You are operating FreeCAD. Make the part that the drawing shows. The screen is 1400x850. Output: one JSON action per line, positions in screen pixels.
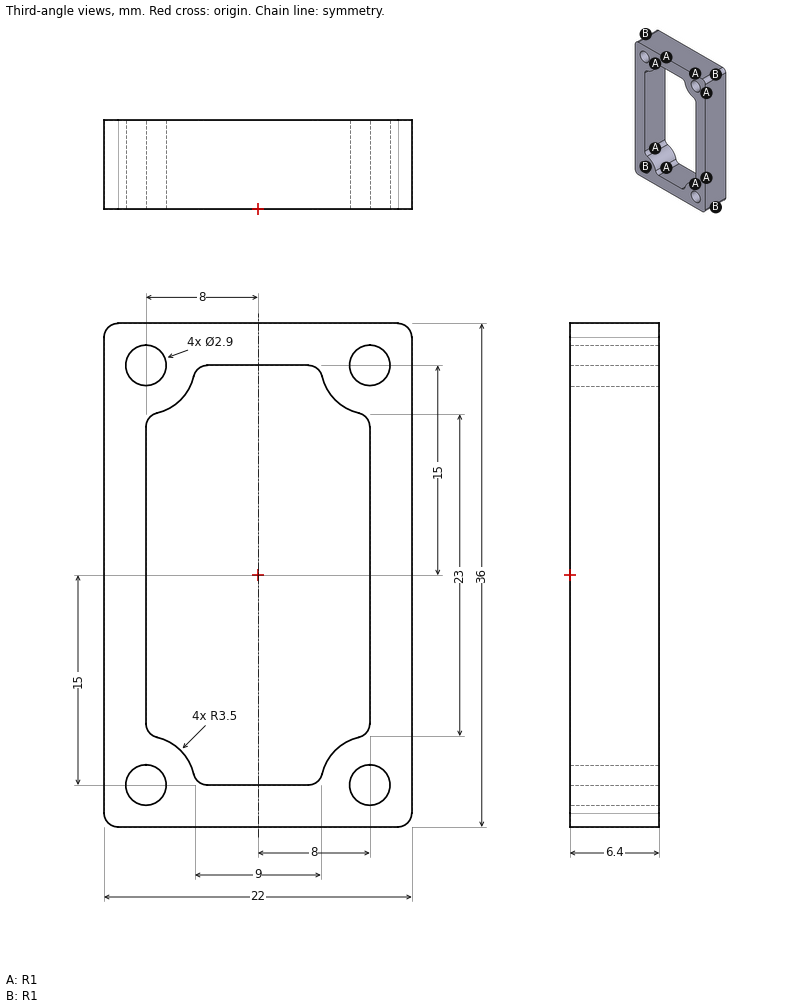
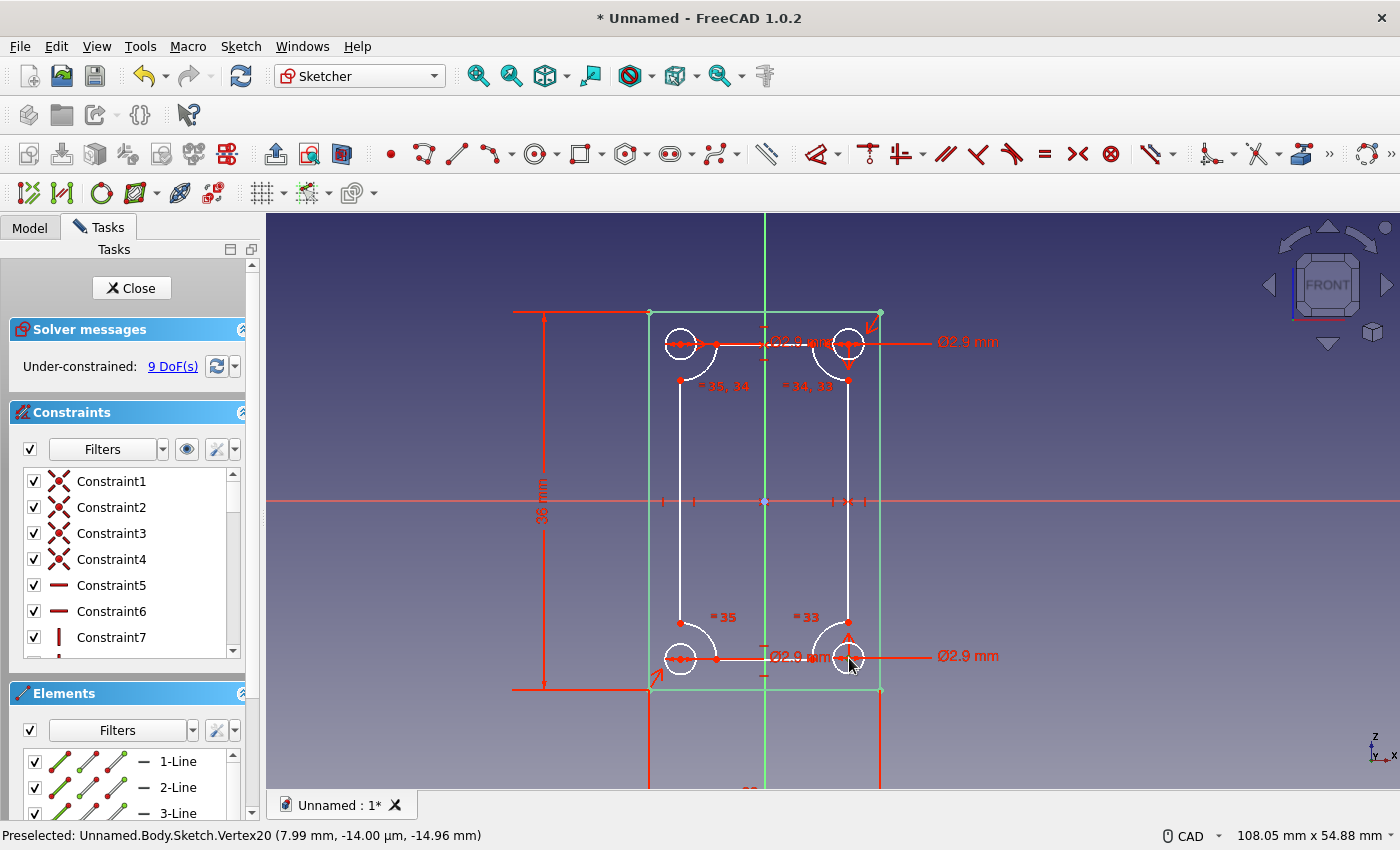
{"action": "left_click", "coordinate": [680, 659]}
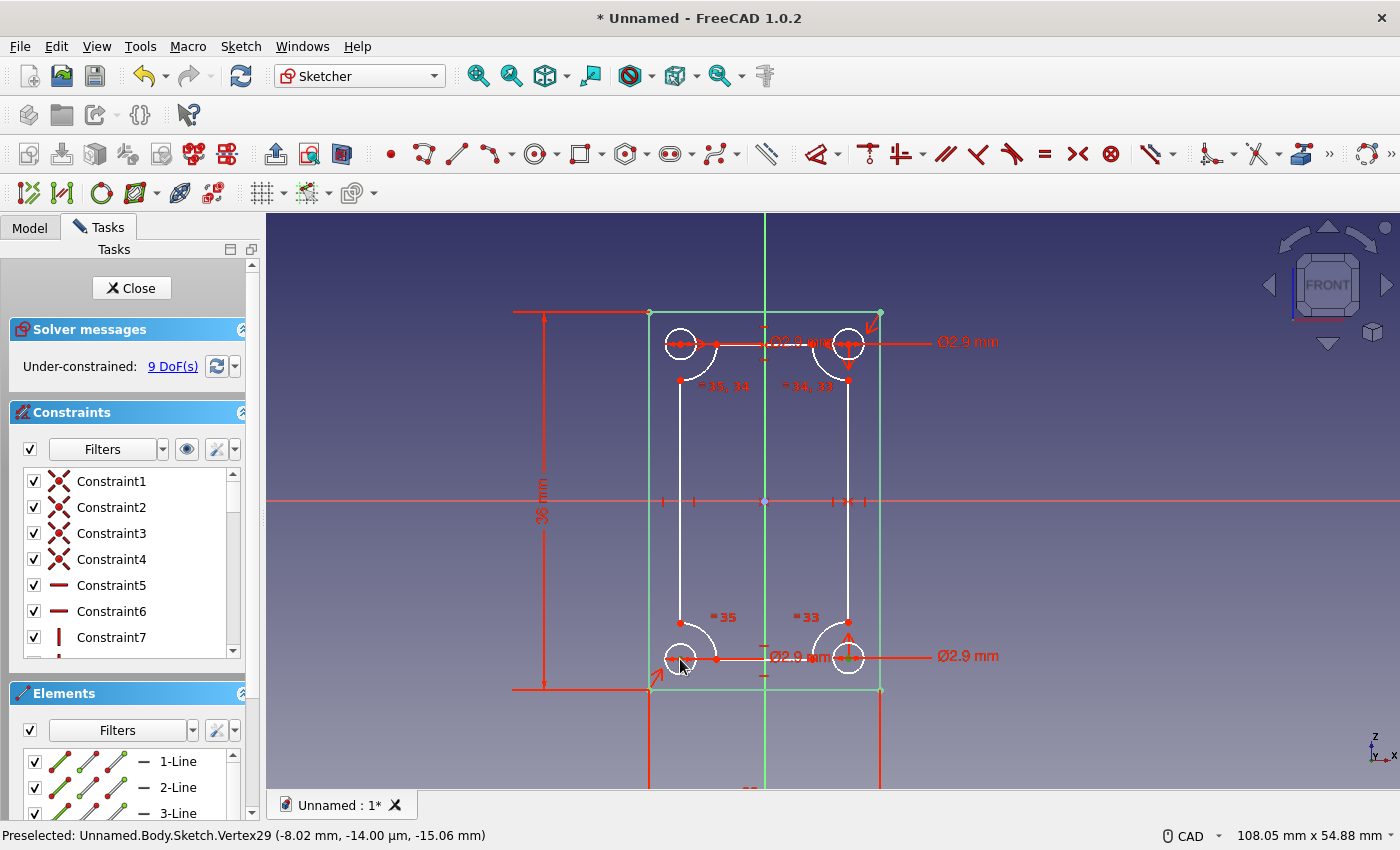
{"action": "left_click", "coordinate": [765, 724]}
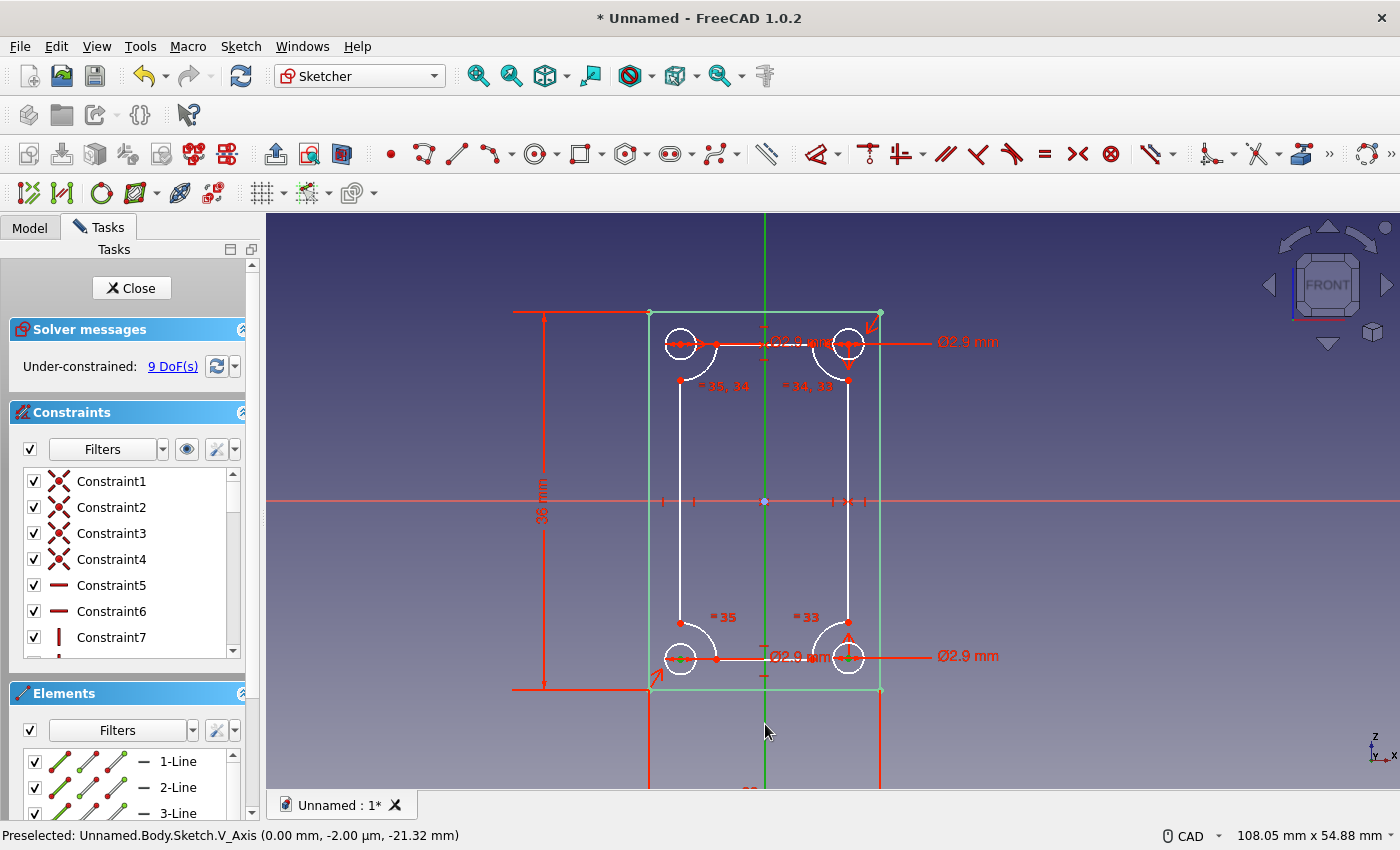
{"action": "left_click", "coordinate": [1078, 154]}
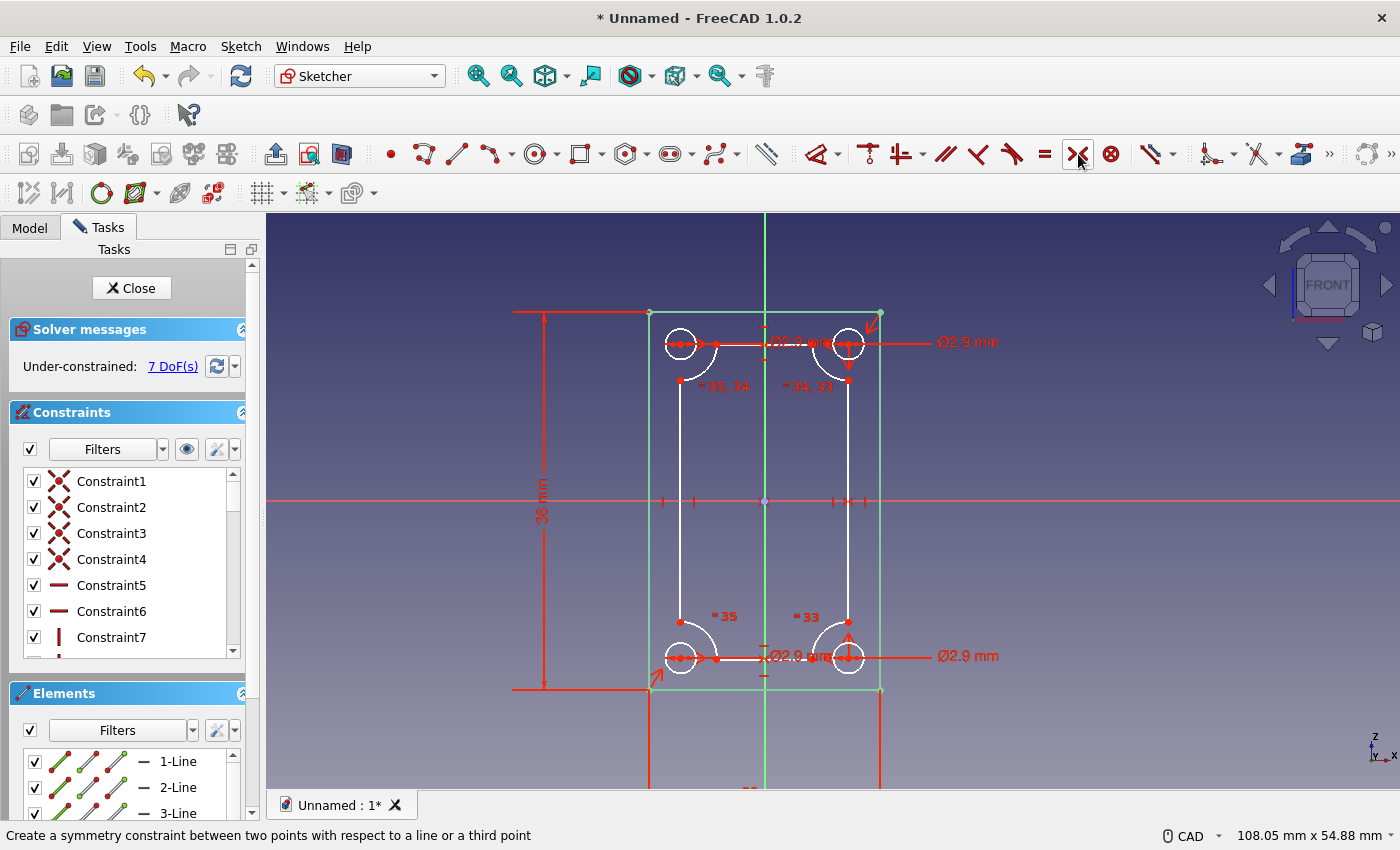
{"action": "left_click", "coordinate": [816, 154]}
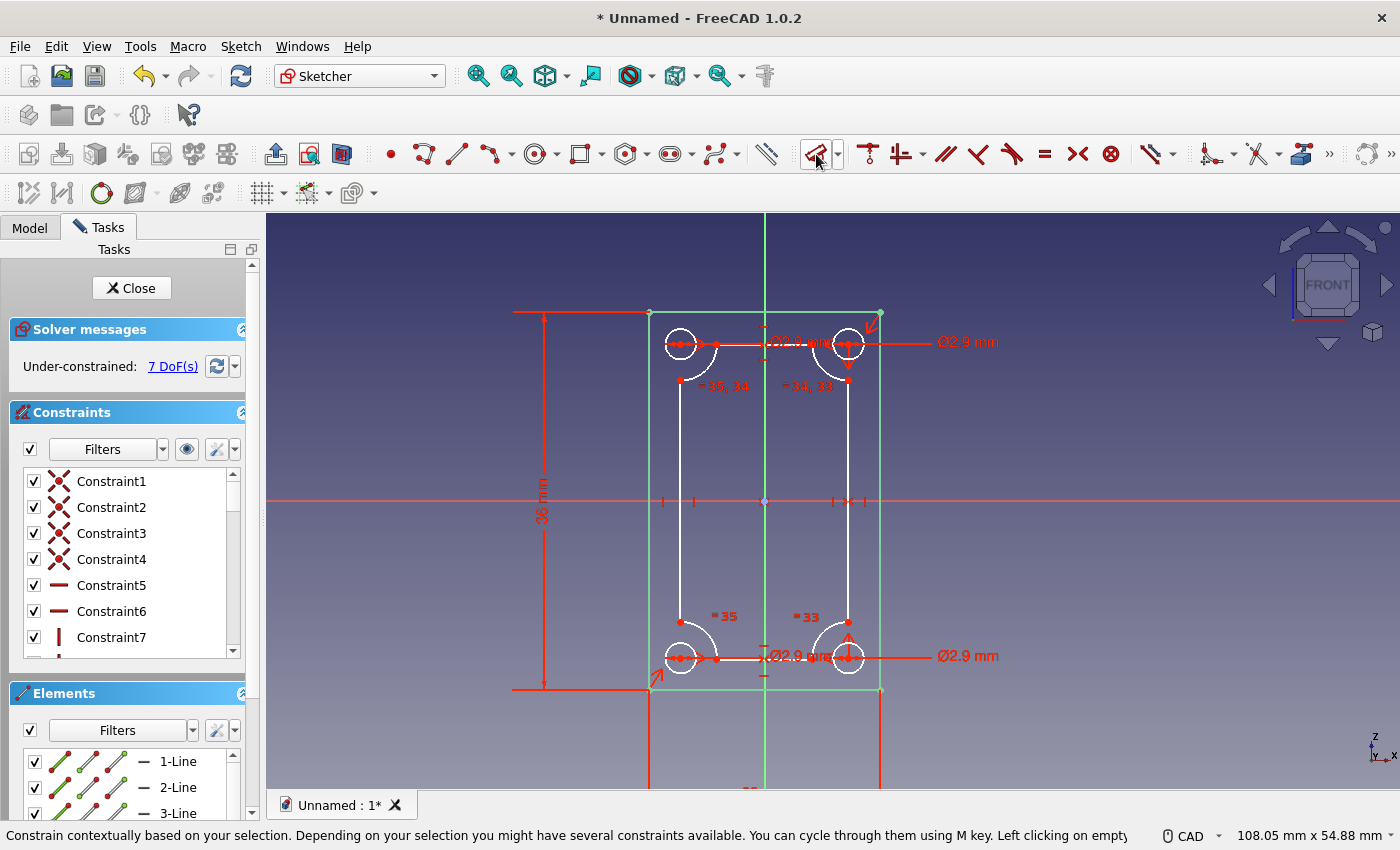
{"action": "left_click", "coordinate": [832, 626]}
{"action": "left_click", "coordinate": [817, 598]}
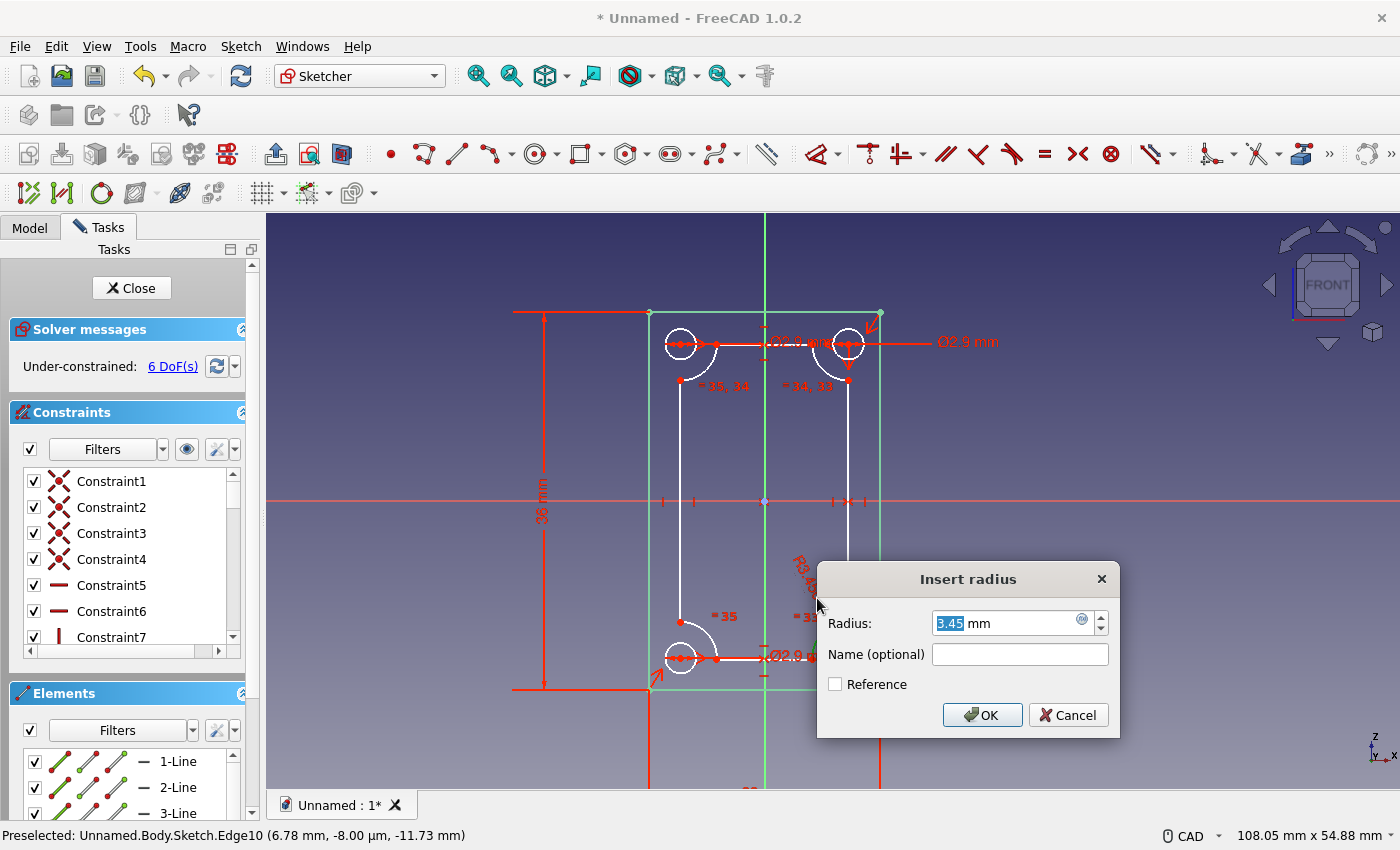
{"action": "type", "text": "3.5"}
{"action": "key", "text": "Return"}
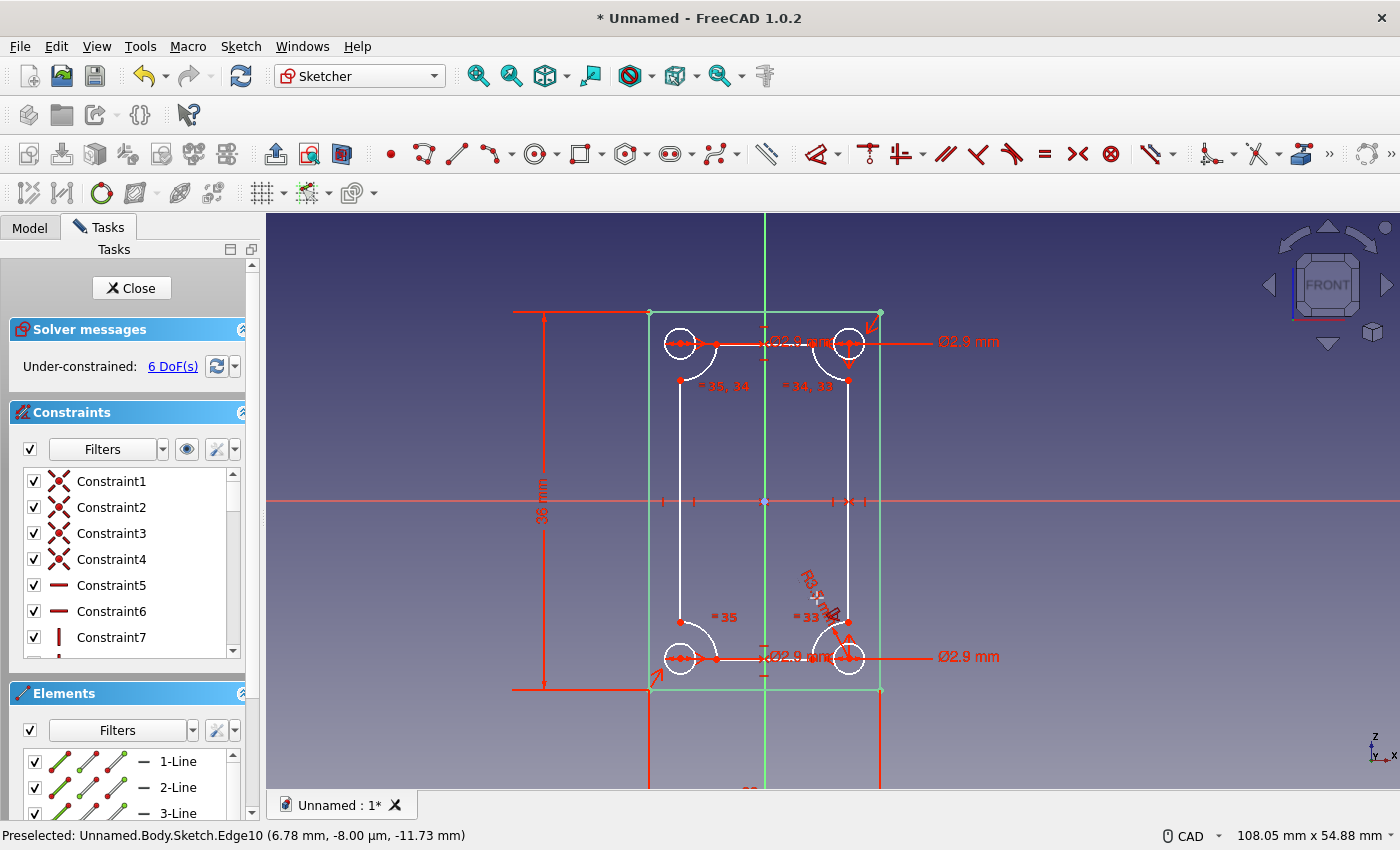
{"action": "left_click", "coordinate": [746, 660]}
{"action": "left_click", "coordinate": [743, 626]}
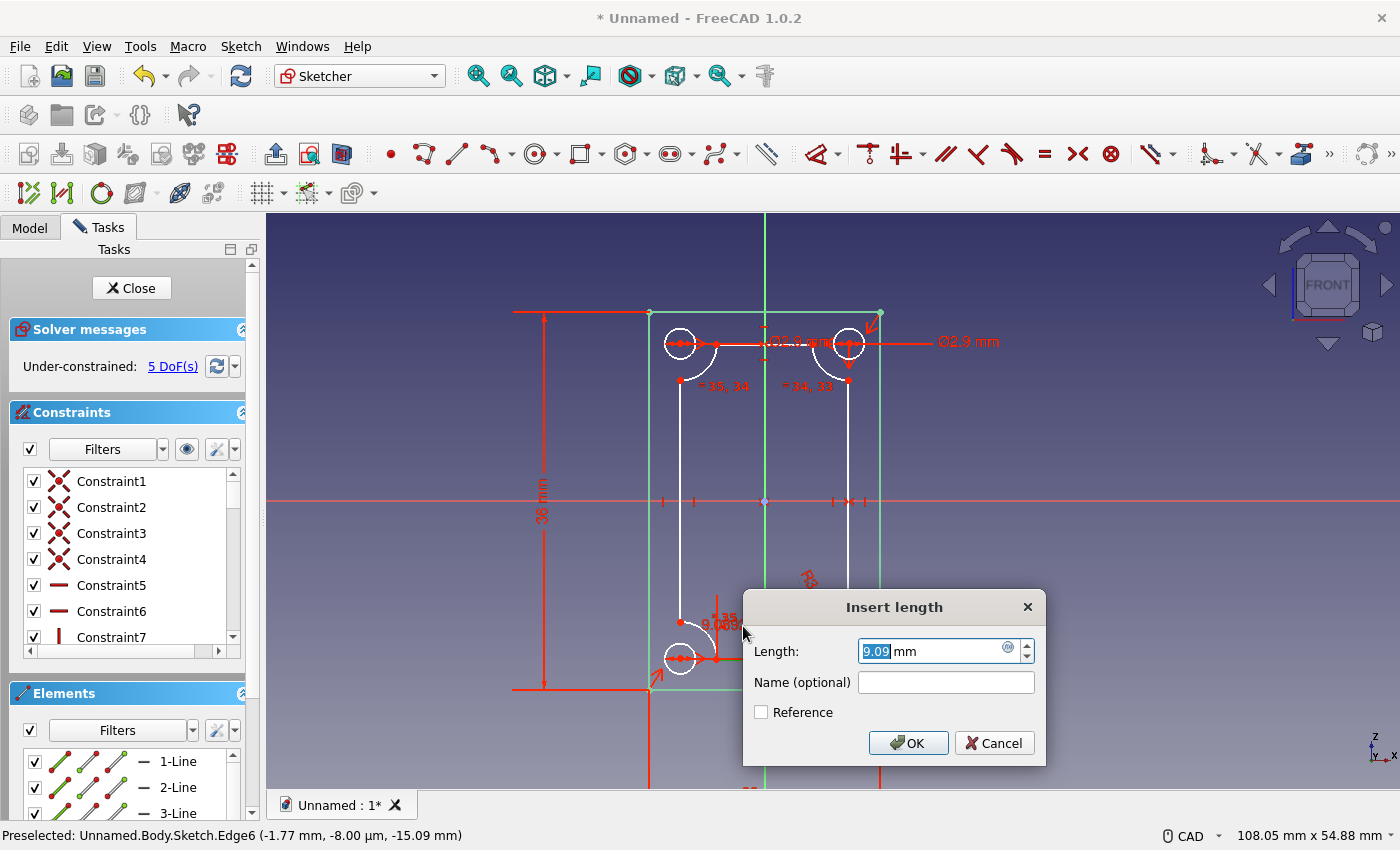
{"action": "type", "text": "9"}
{"action": "key", "text": "Return"}